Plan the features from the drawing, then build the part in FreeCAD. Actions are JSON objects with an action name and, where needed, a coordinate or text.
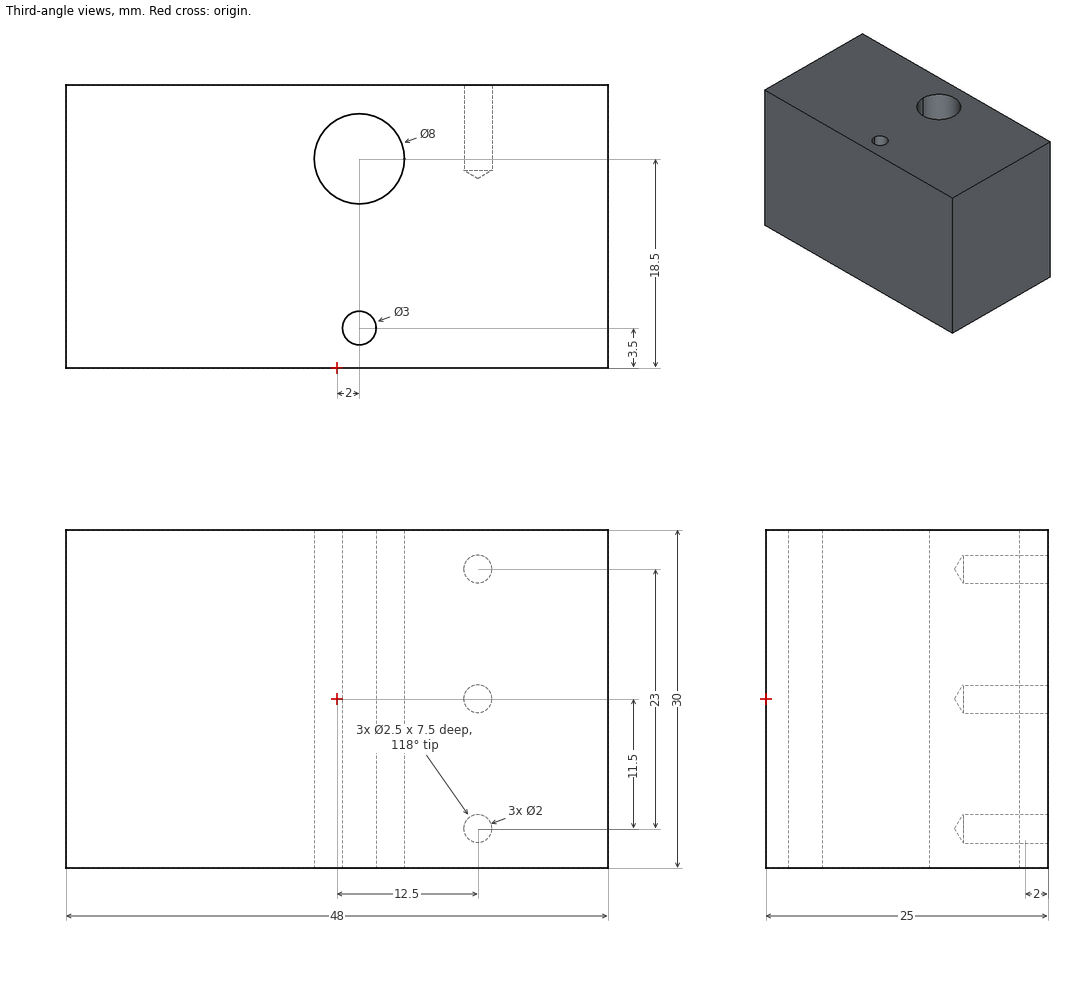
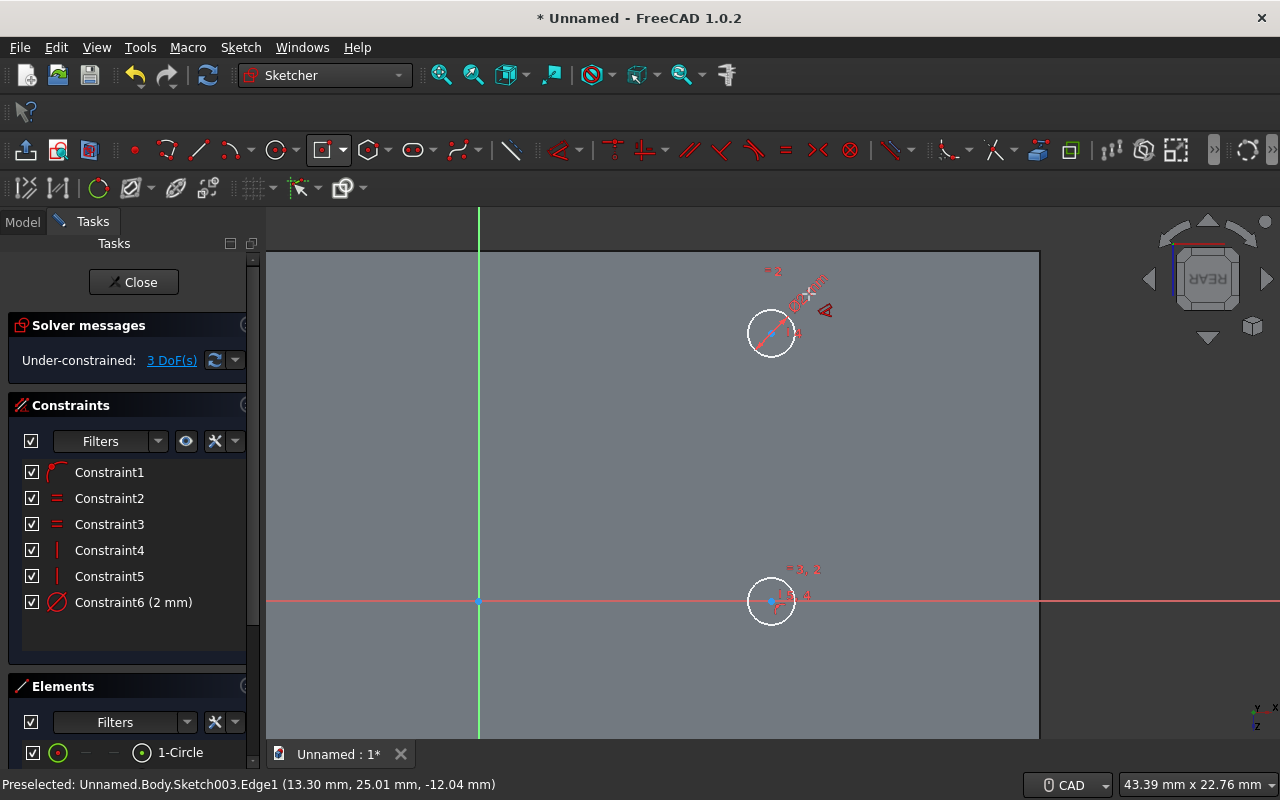
{"action": "left_click", "coordinate": [771, 333]}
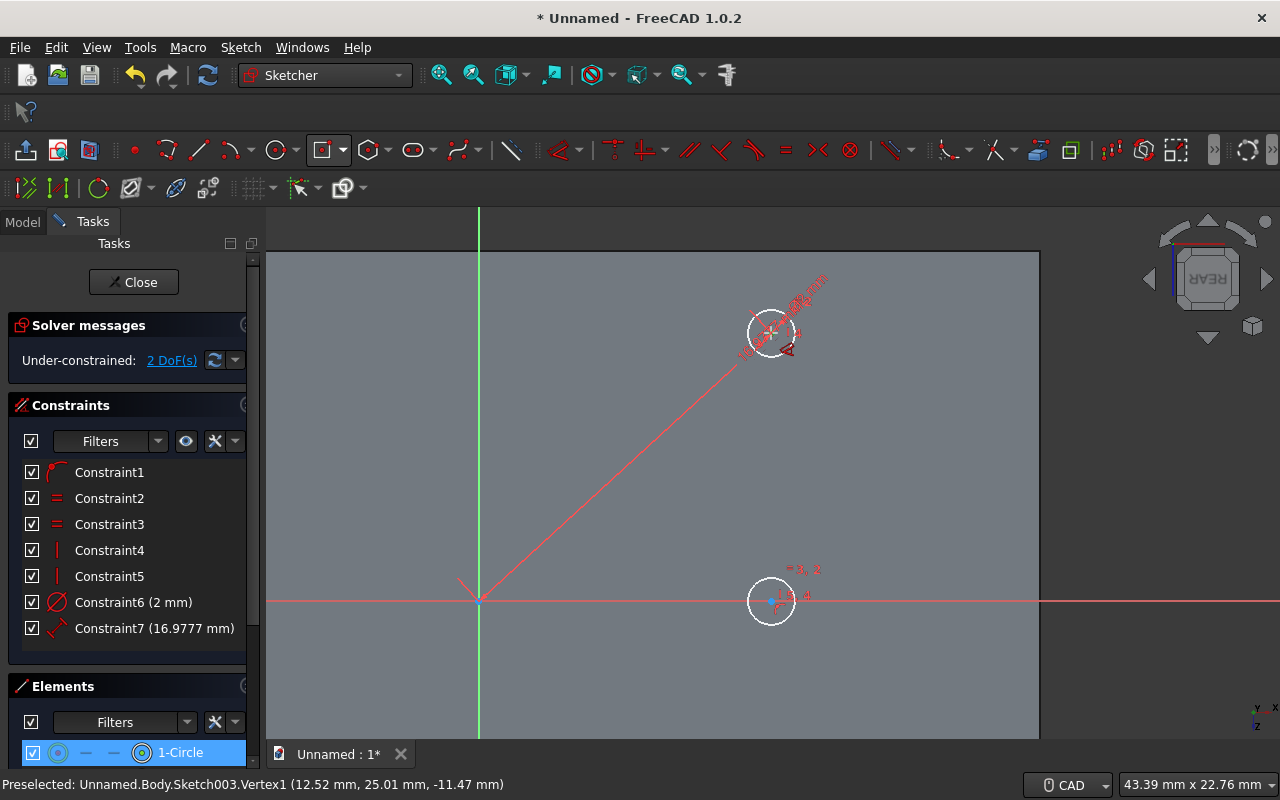
{"action": "scroll", "coordinate": [787, 317], "scroll_direction": "down", "scroll_amount": 3}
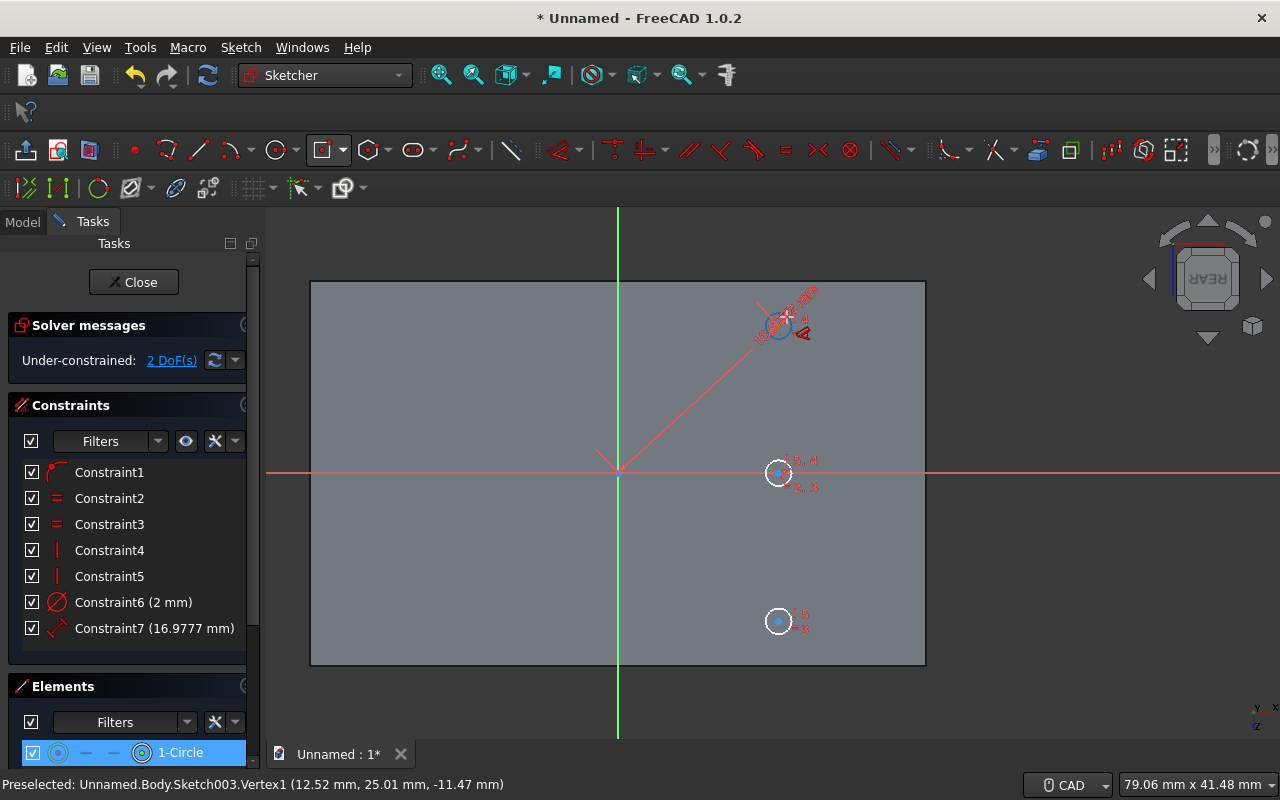
{"action": "left_click", "coordinate": [779, 621]}
{"action": "left_click", "coordinate": [813, 406]}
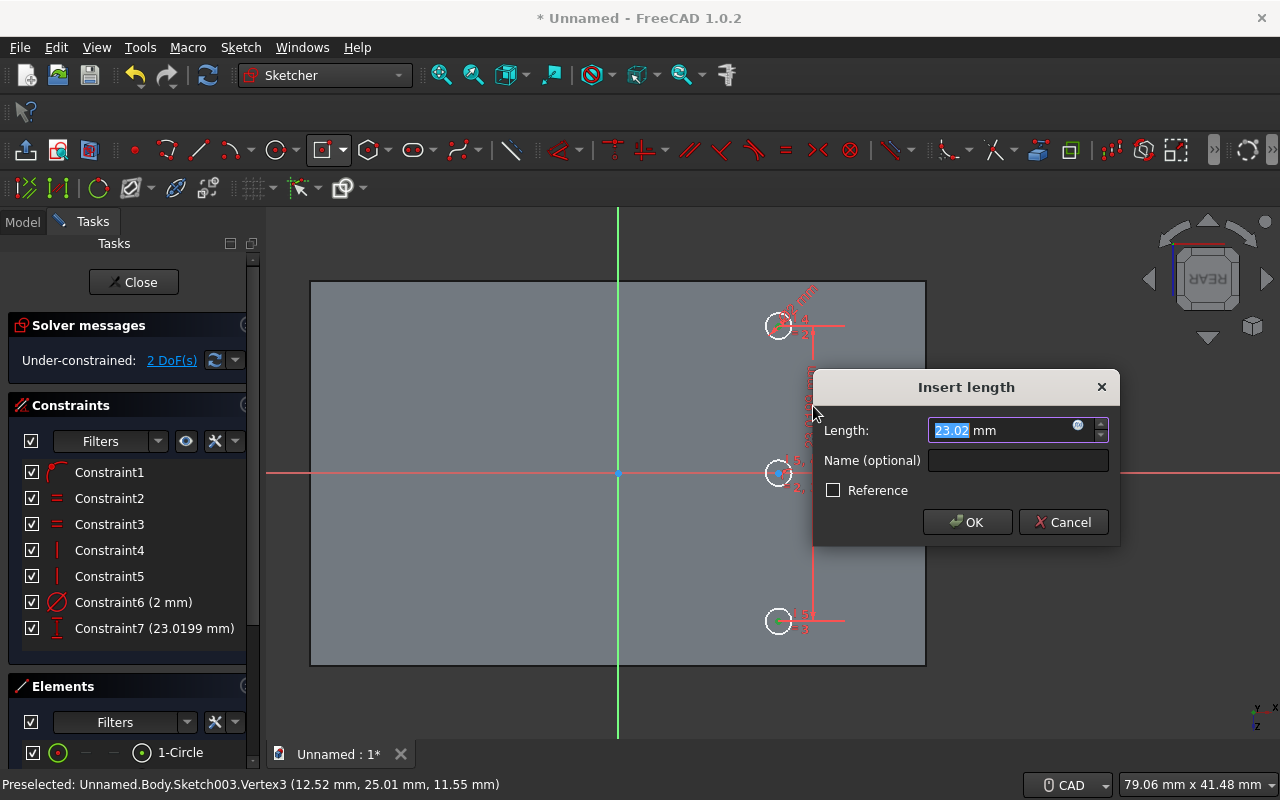
{"action": "type", "text": "23"}
{"action": "key", "text": "Return"}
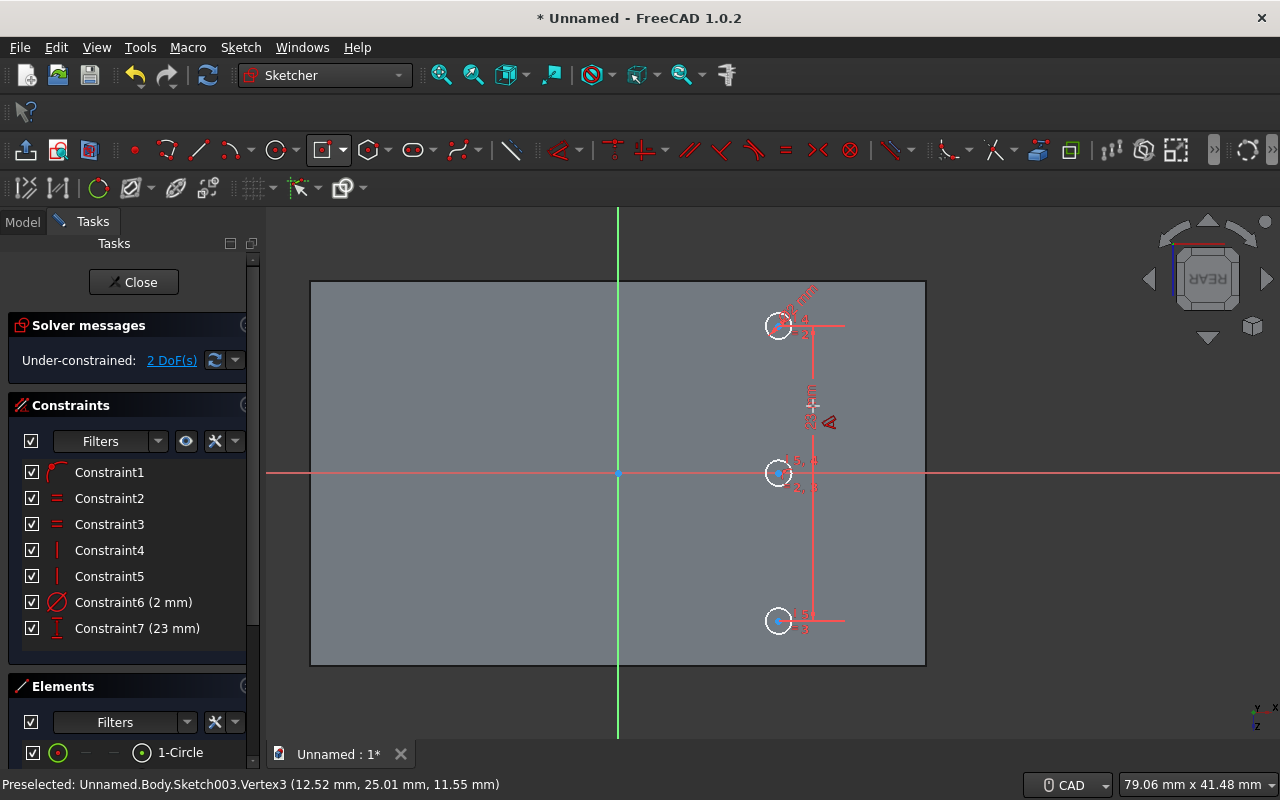
{"action": "left_click", "coordinate": [779, 326]}
{"action": "left_click", "coordinate": [698, 292]}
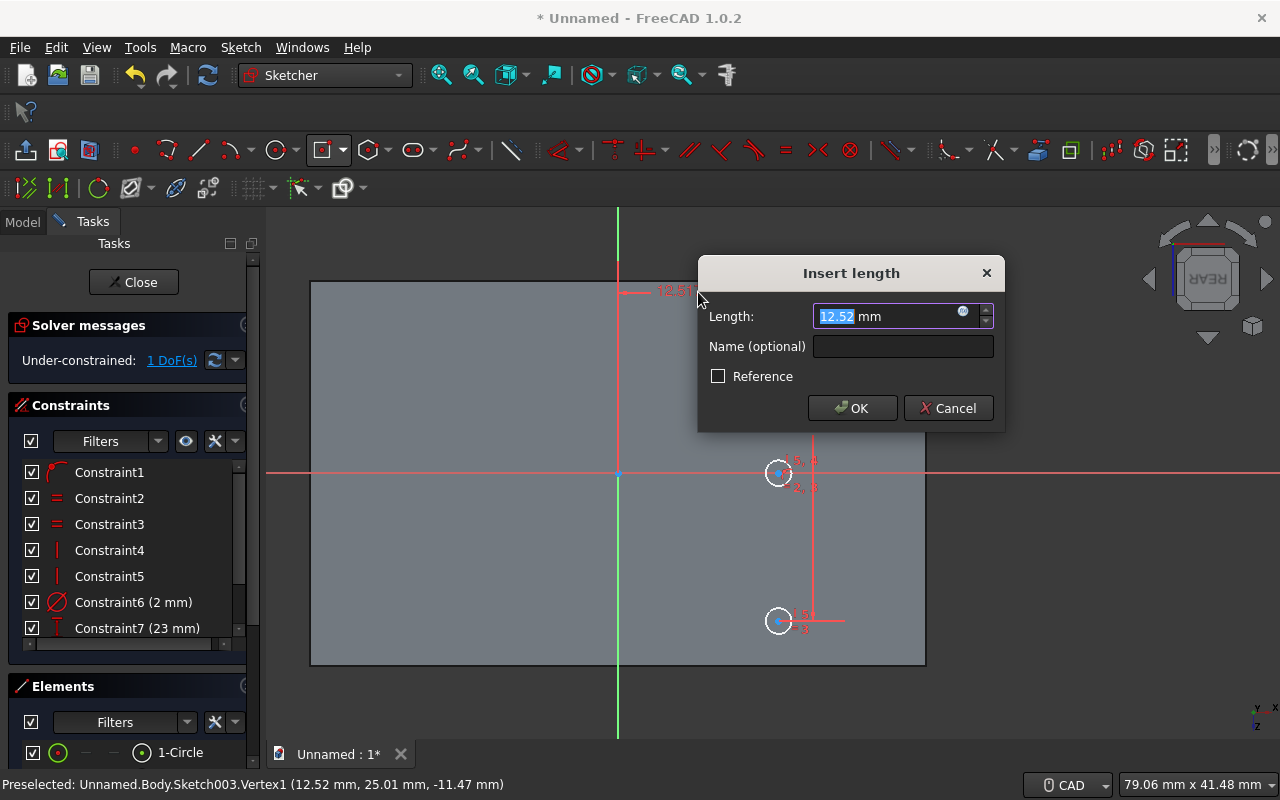
{"action": "type", "text": "12.5"}
{"action": "key", "text": "Return"}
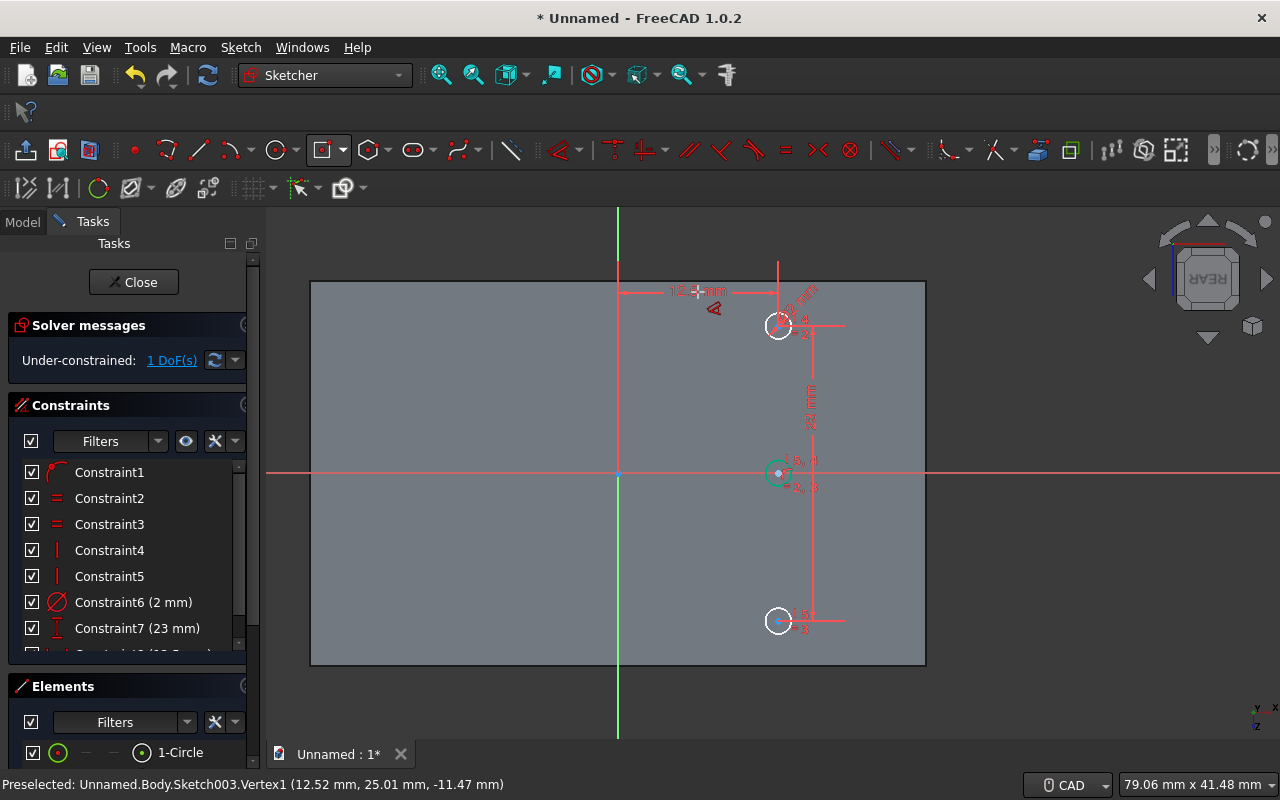
{"action": "left_click", "coordinate": [778, 326]}
{"action": "left_click", "coordinate": [584, 400]}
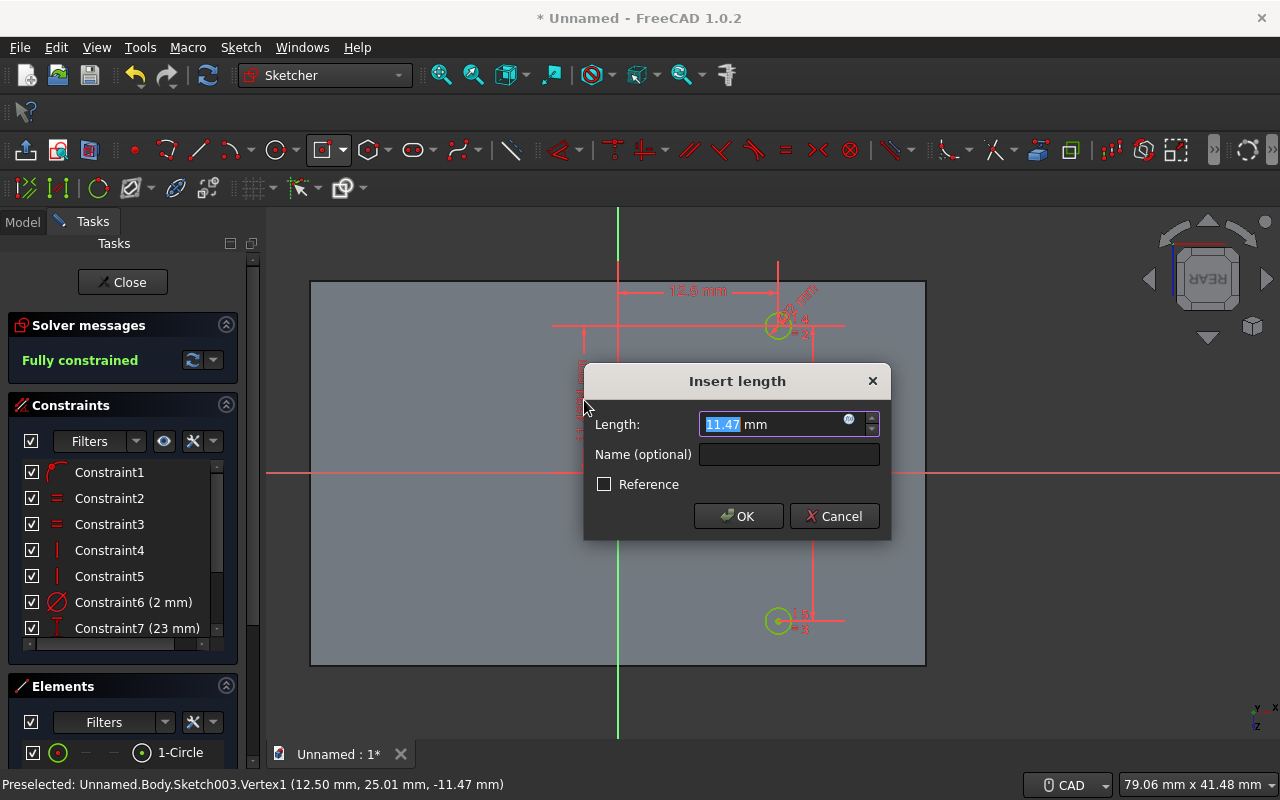
{"action": "type", "text": "11.5"}
{"action": "key", "text": "Return"}
{"action": "key", "text": "Escape"}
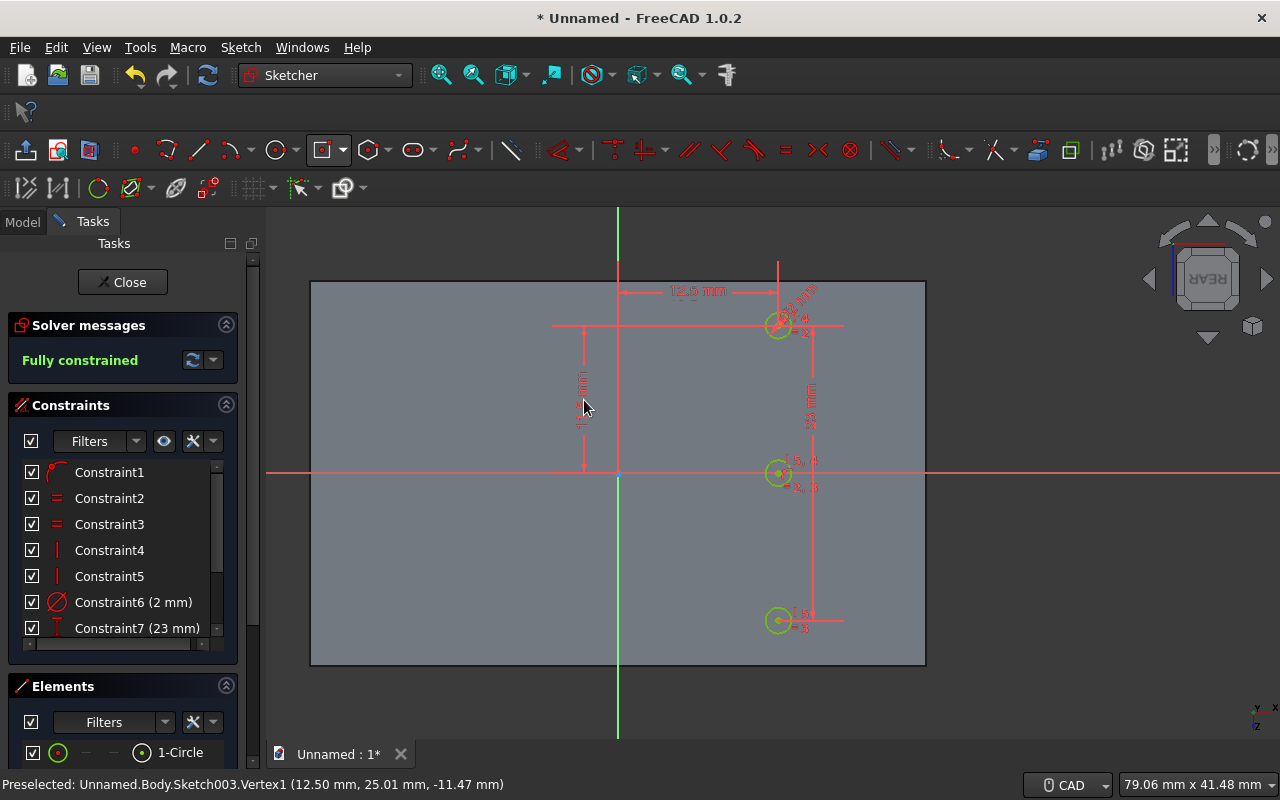
{"action": "left_click", "coordinate": [123, 282]}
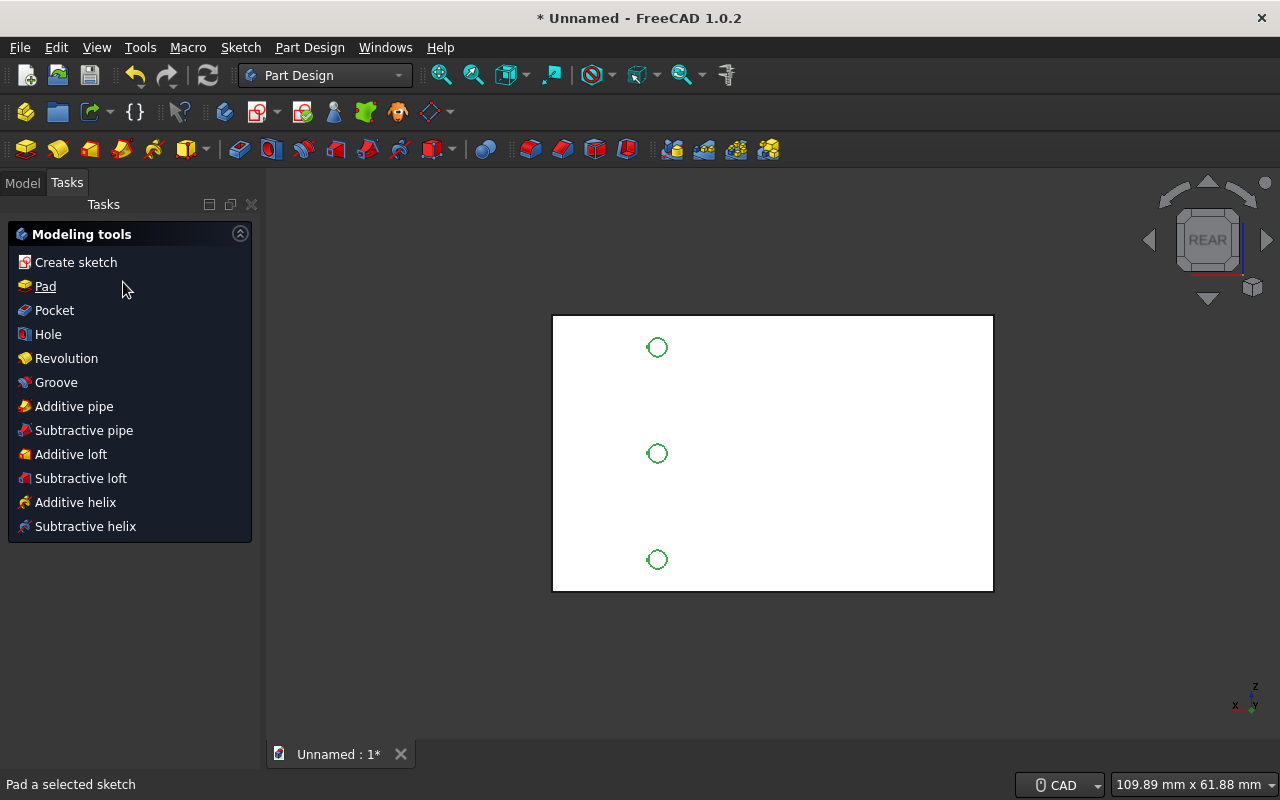
{"action": "left_click", "coordinate": [240, 150]}